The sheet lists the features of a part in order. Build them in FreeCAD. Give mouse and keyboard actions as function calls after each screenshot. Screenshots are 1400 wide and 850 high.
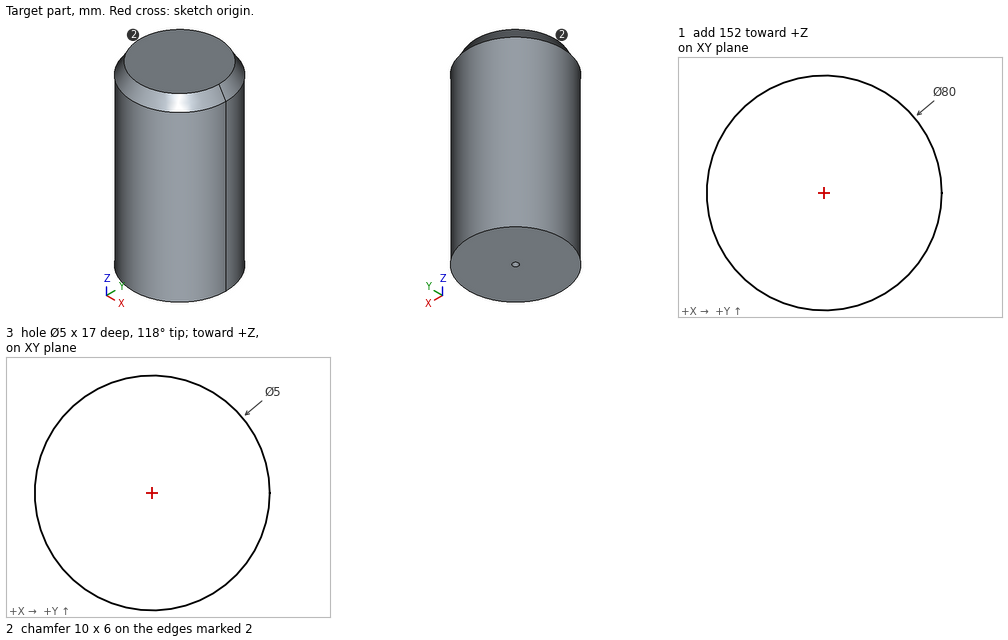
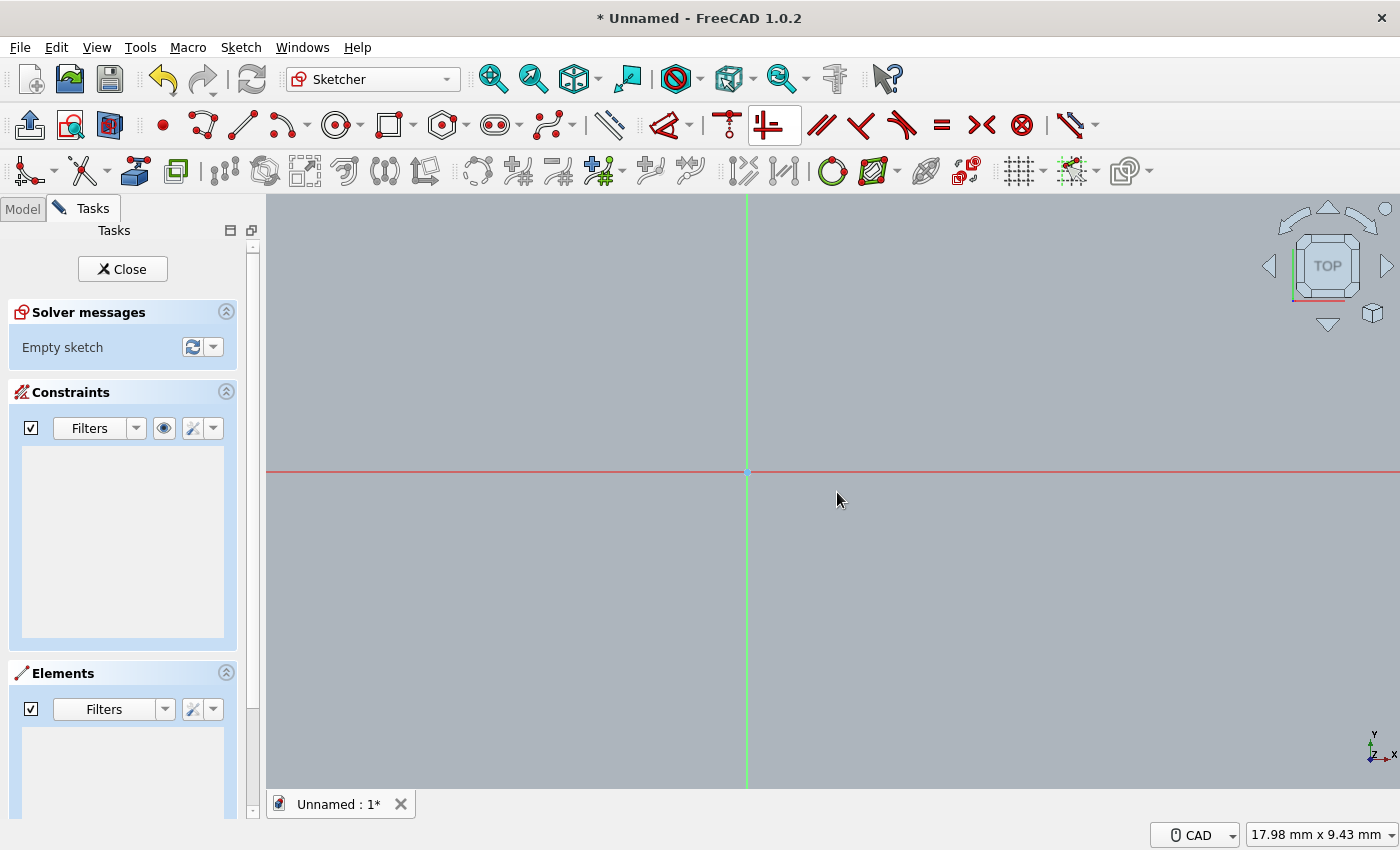
click(336, 126)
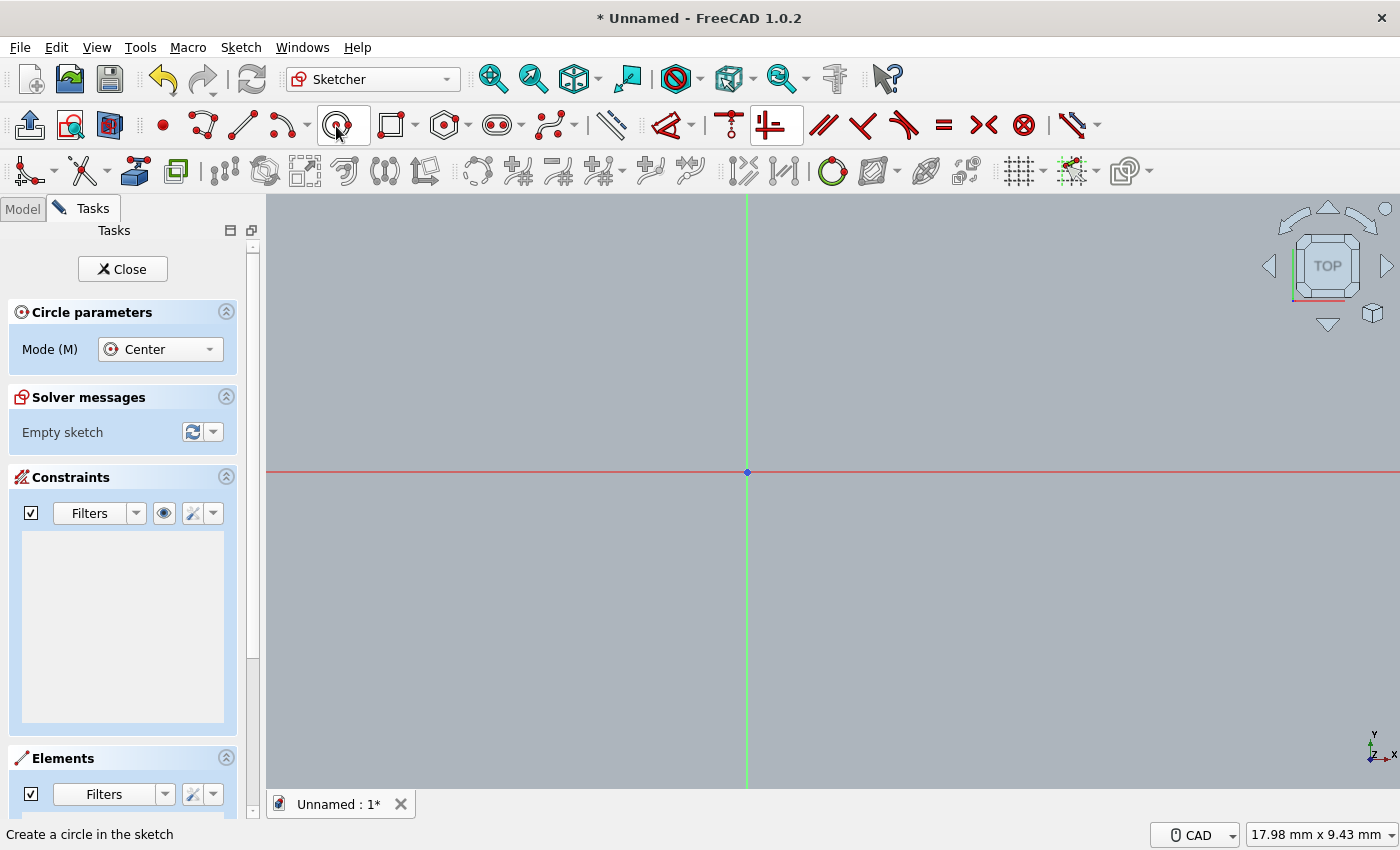
click(747, 472)
click(859, 361)
key(Escape)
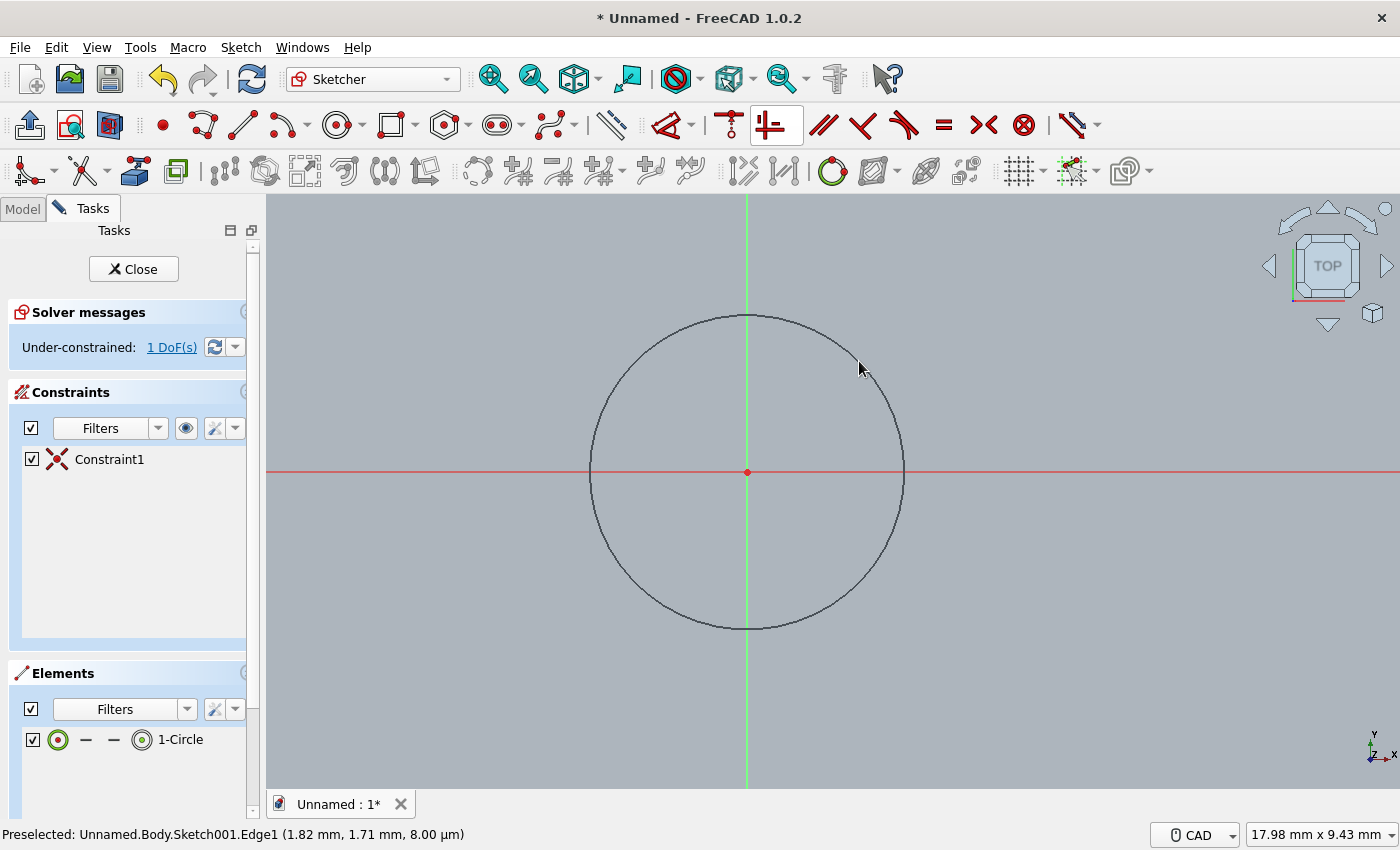
click(666, 126)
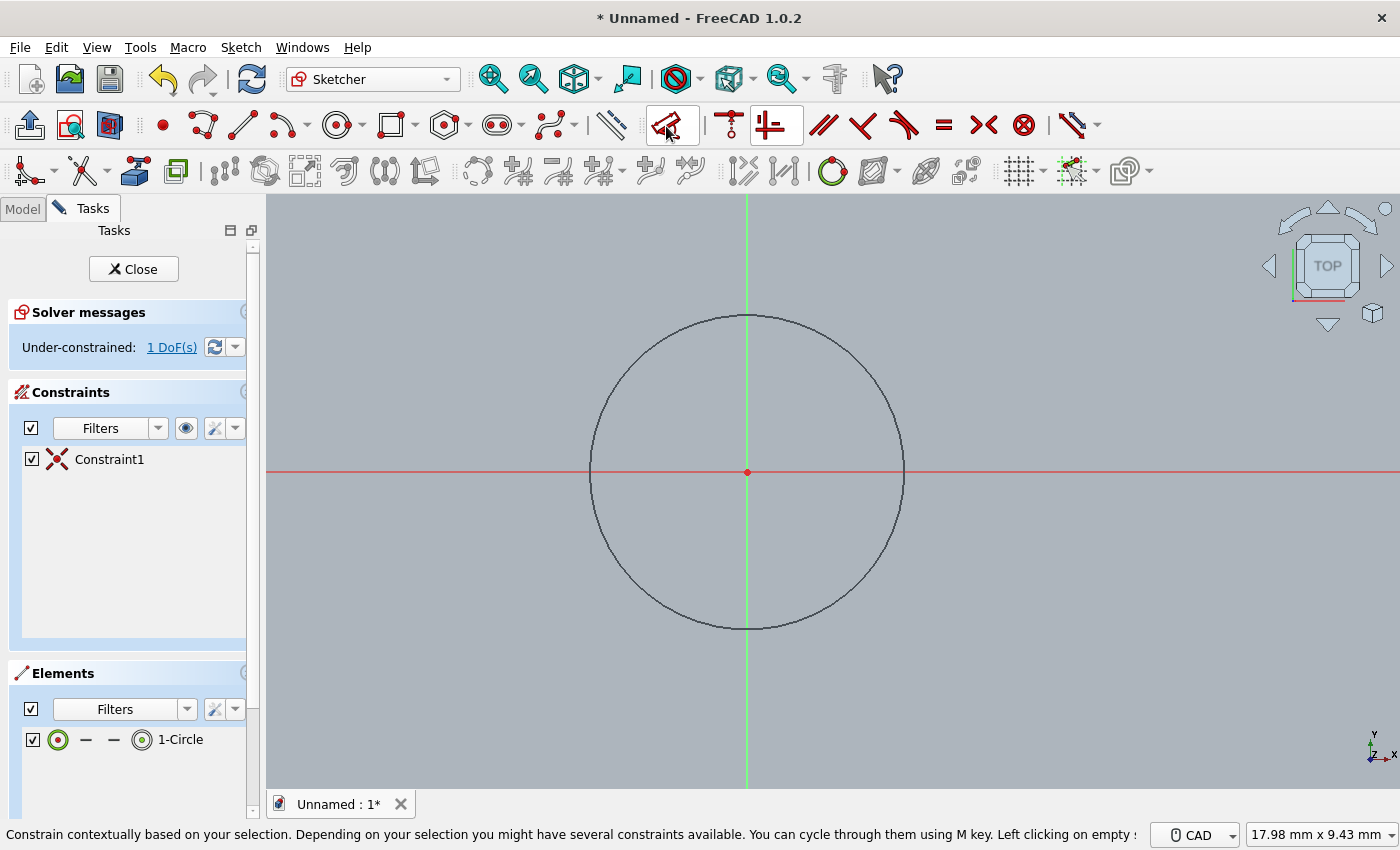
click(858, 361)
click(881, 338)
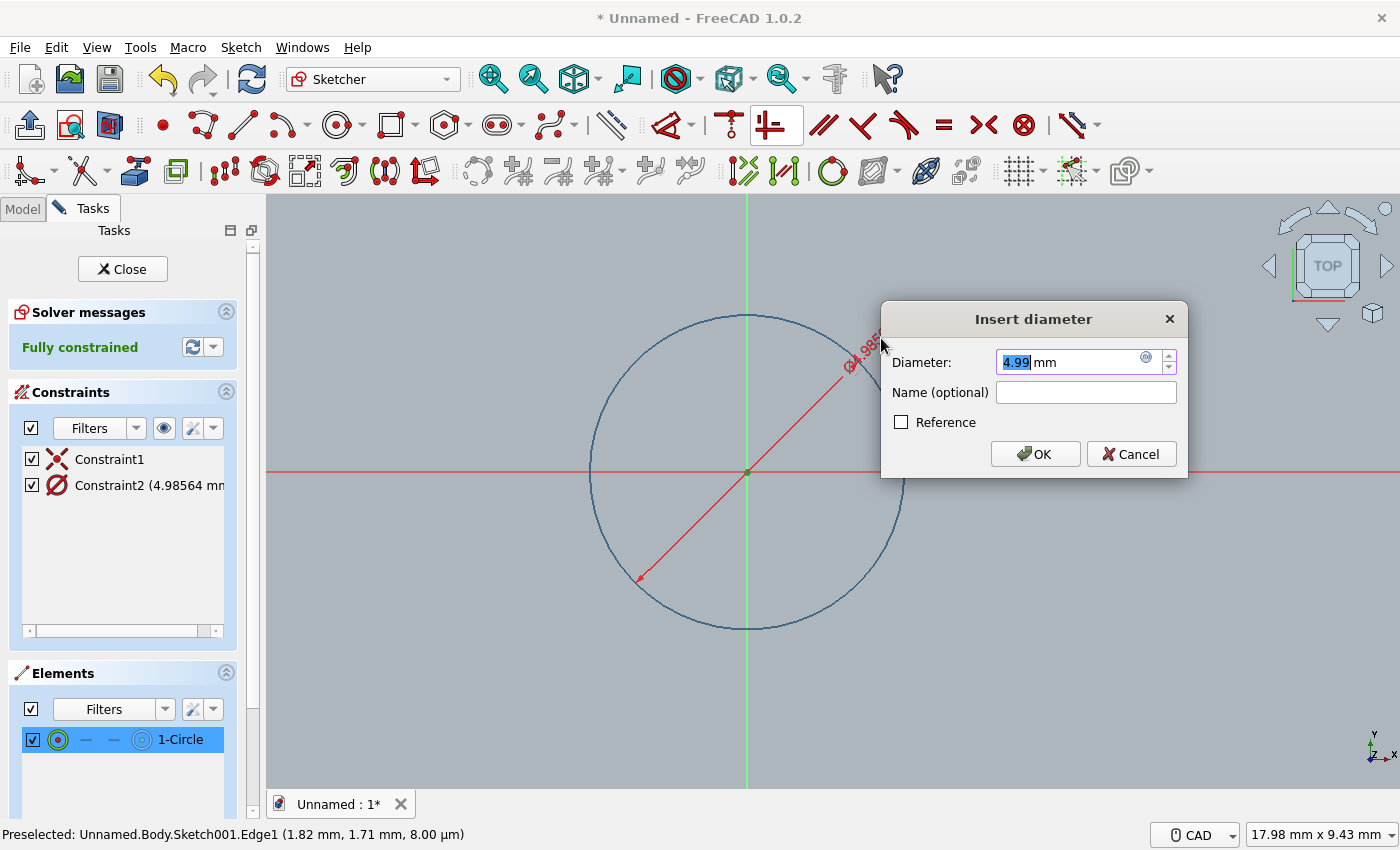
text(5)
key(Return)
key(Escape)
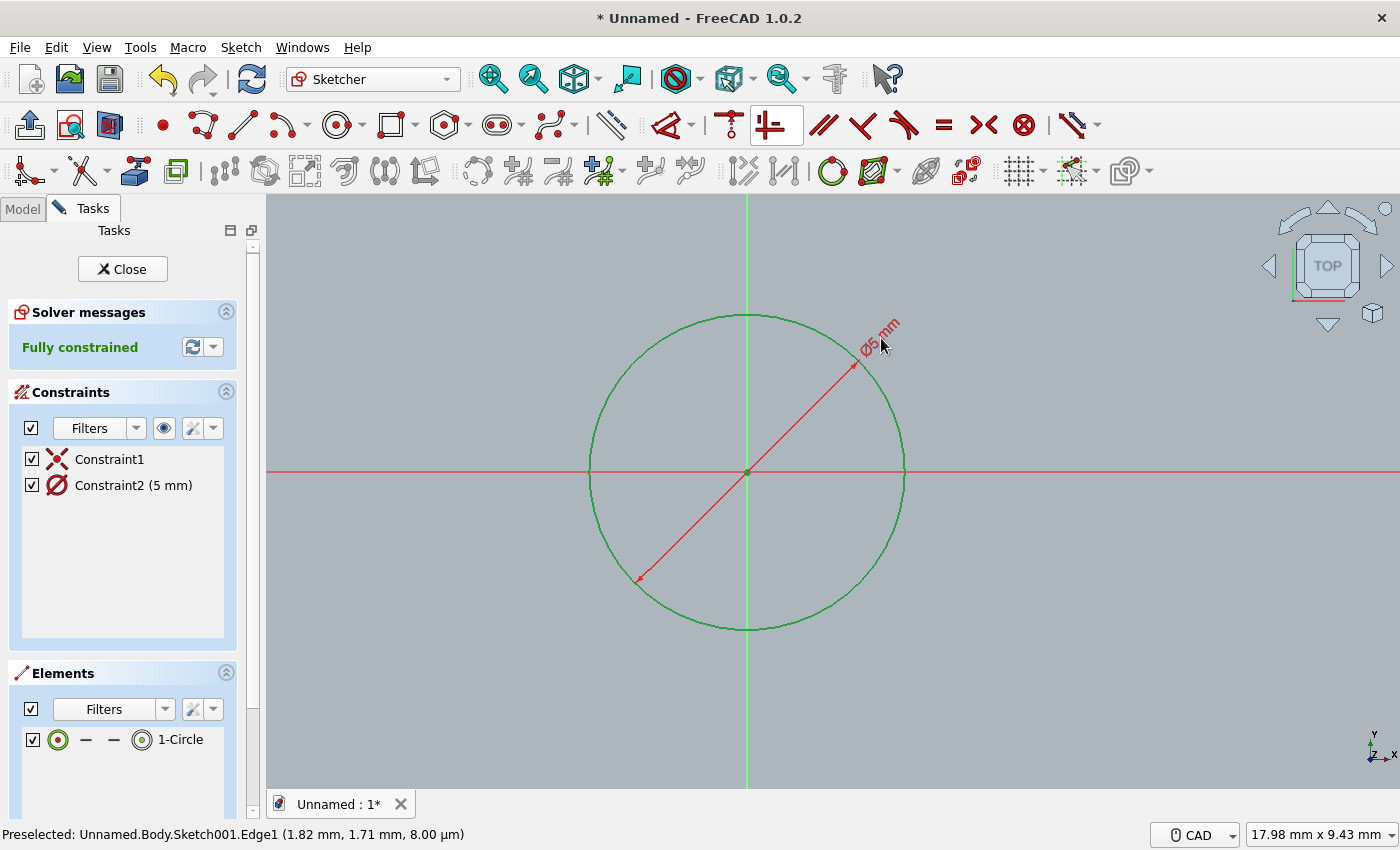
click(123, 269)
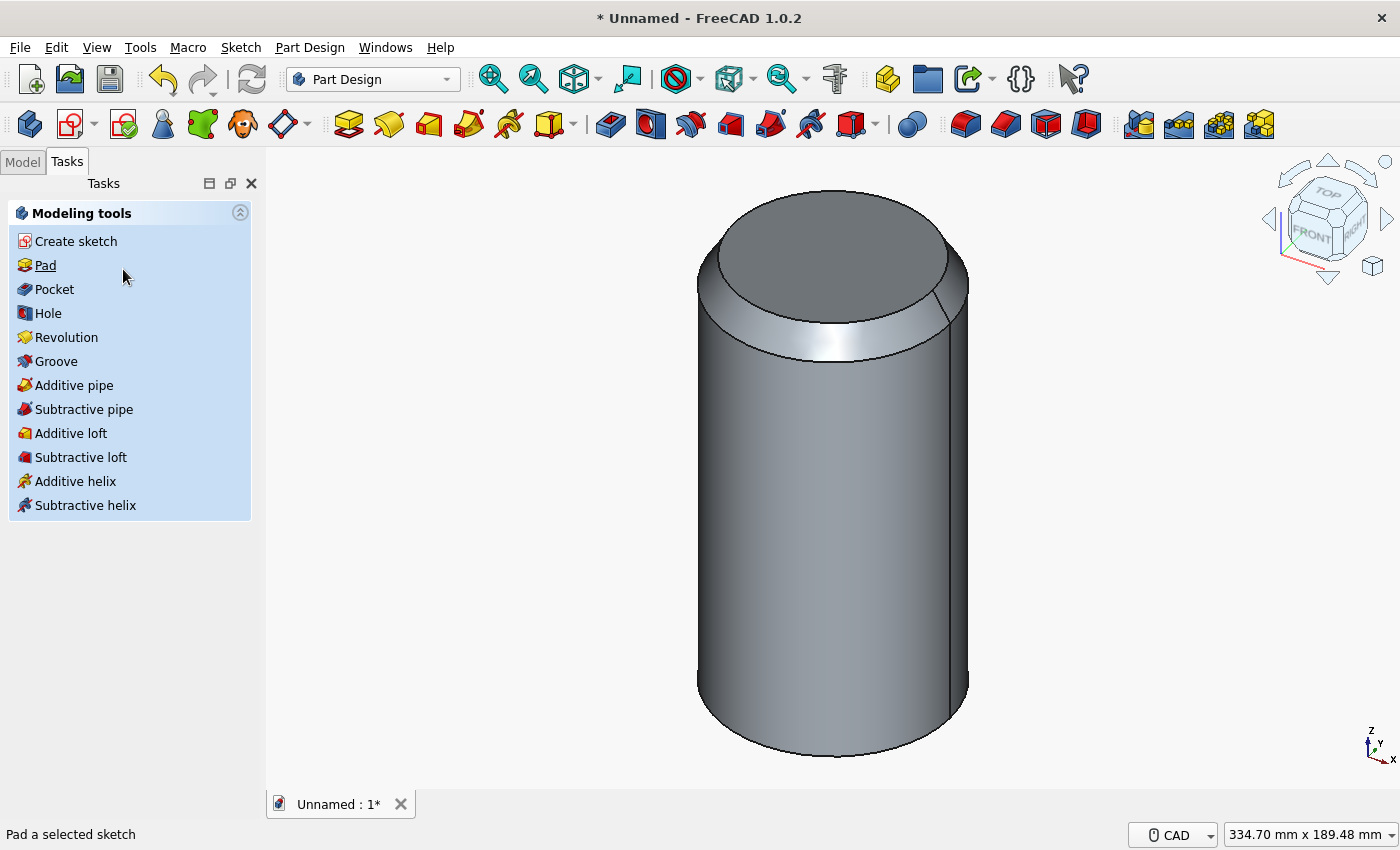
click(652, 124)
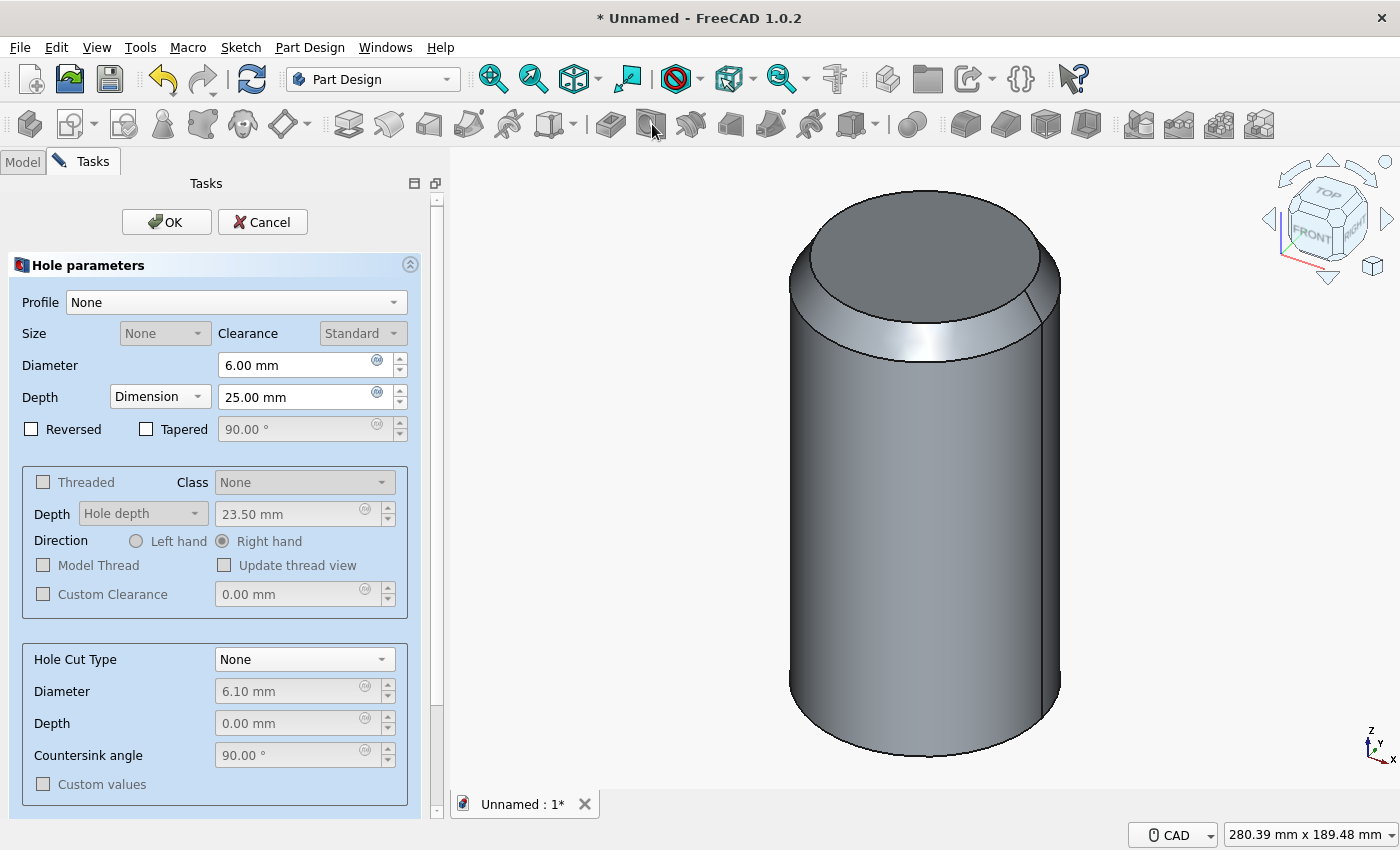
triple_click(305, 365)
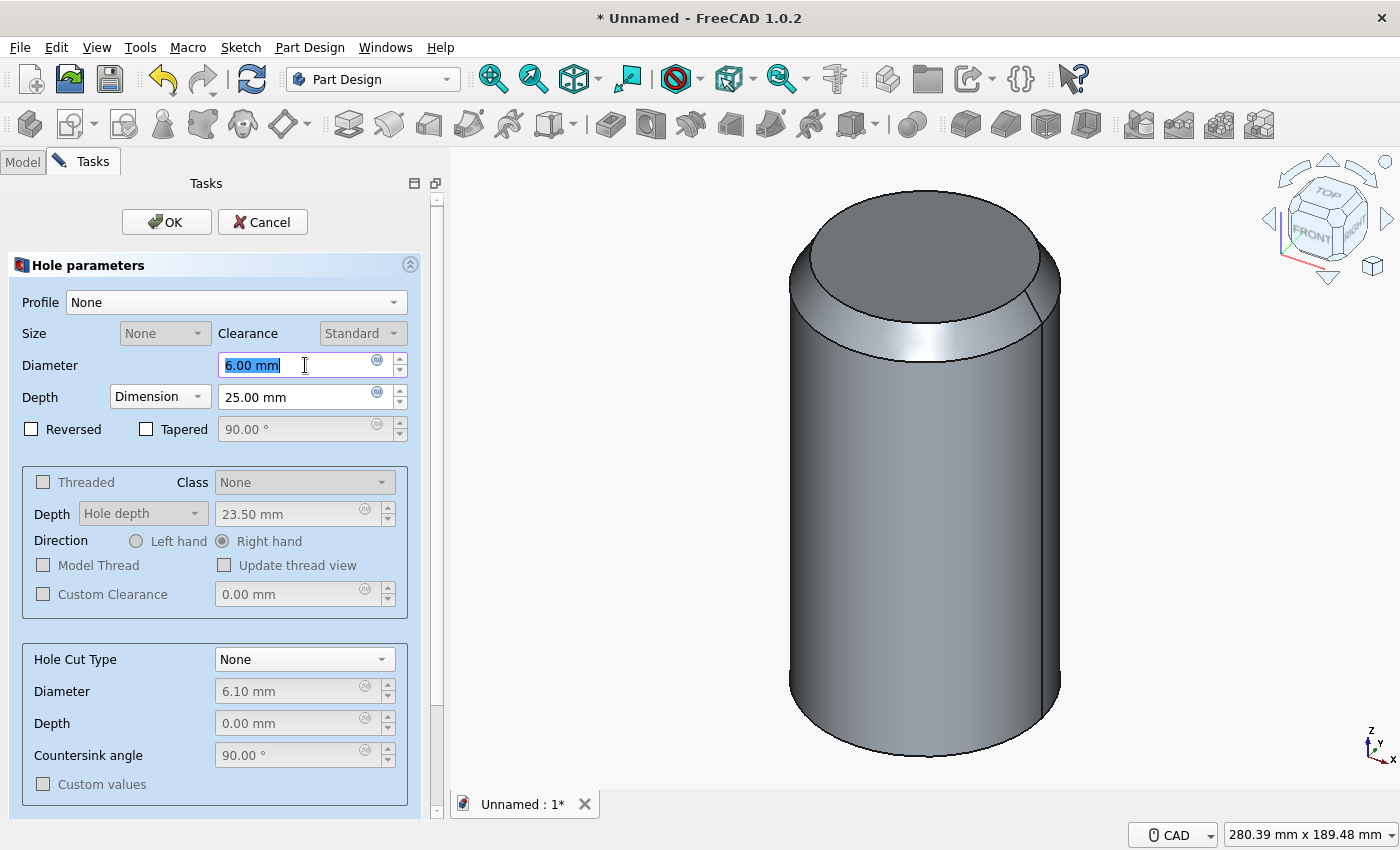
text(5)
key(Tab)